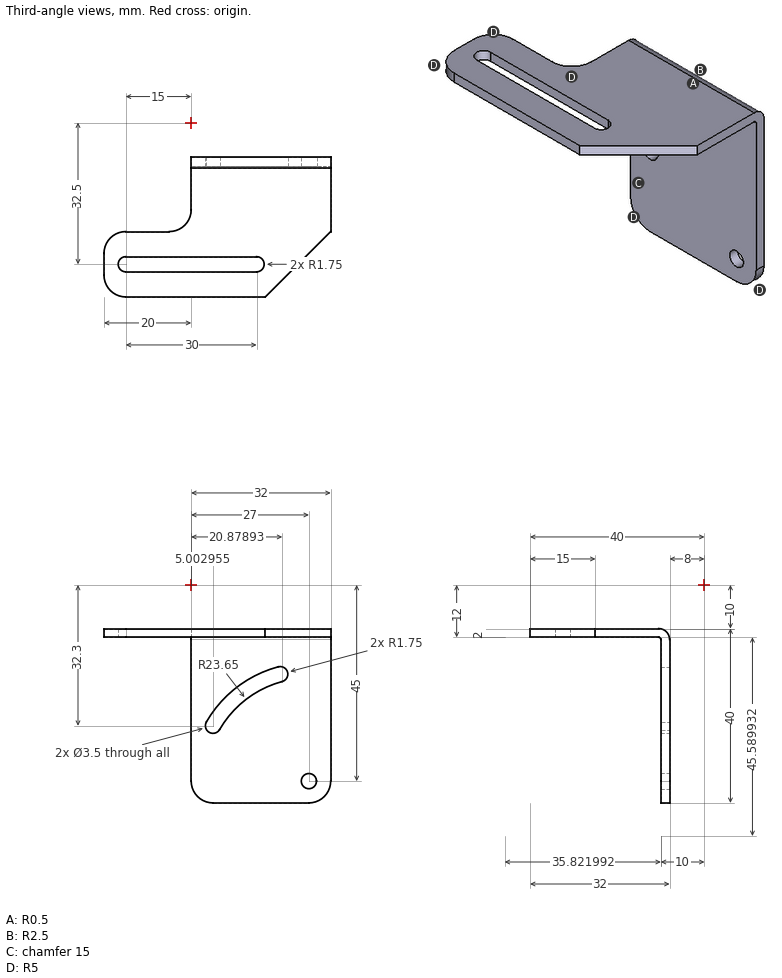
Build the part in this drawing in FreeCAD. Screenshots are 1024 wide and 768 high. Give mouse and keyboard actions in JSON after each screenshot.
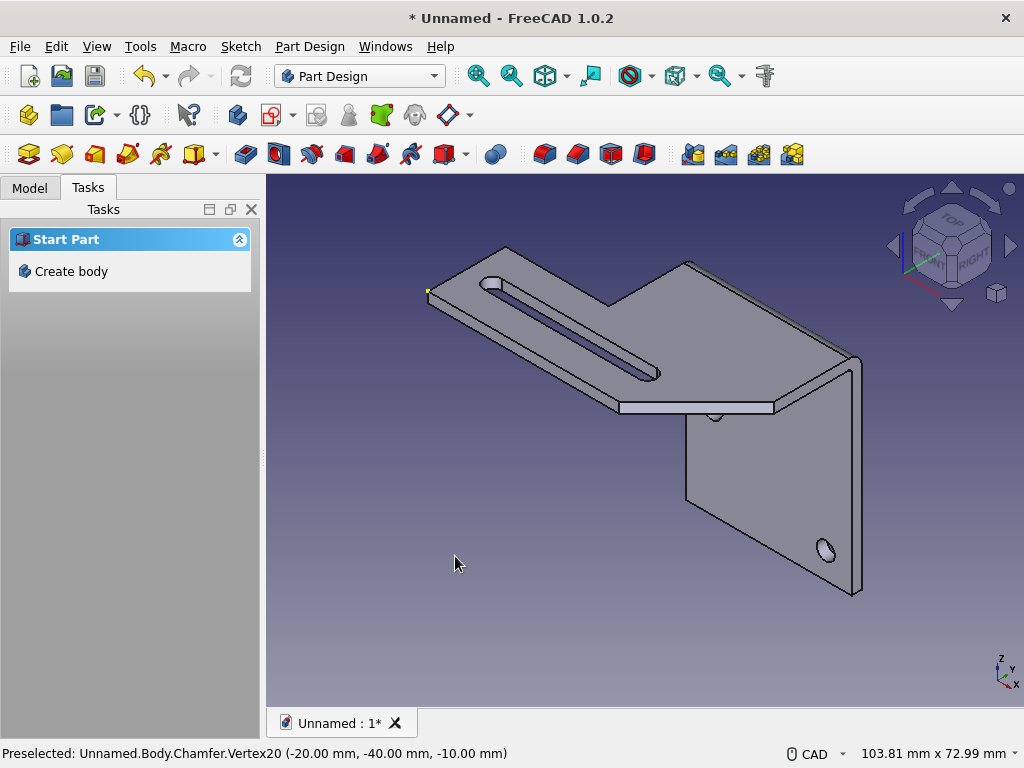
{"action": "scroll", "coordinate": [428, 296], "scroll_direction": "up", "scroll_amount": 6}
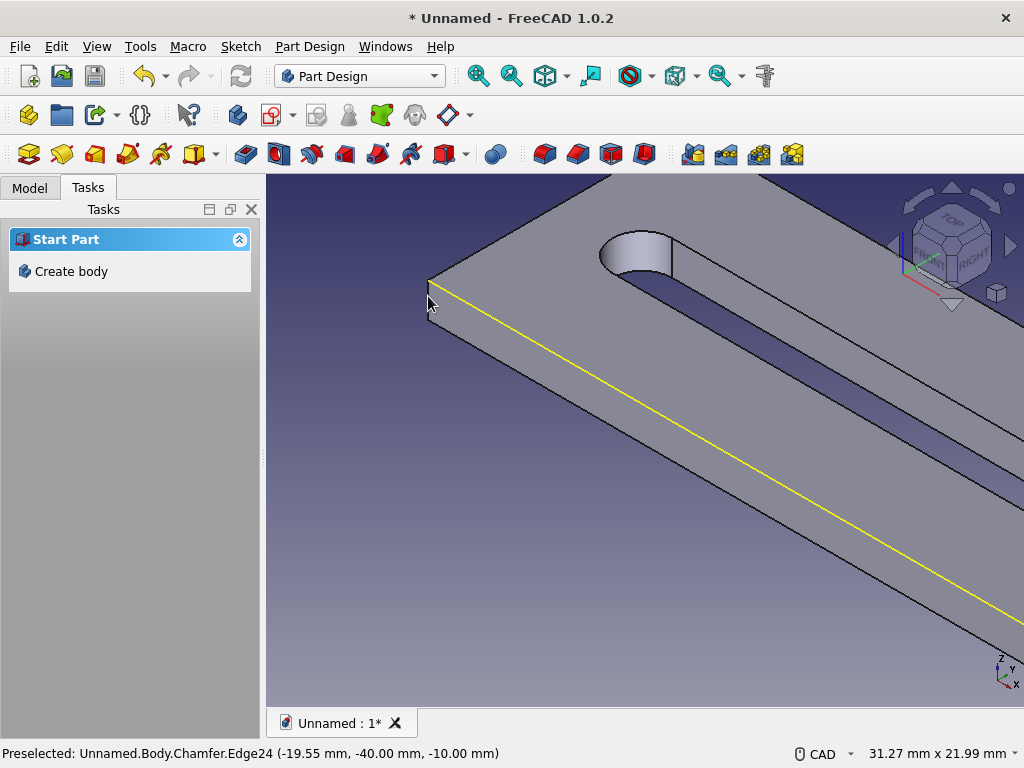
{"action": "left_click", "coordinate": [479, 76]}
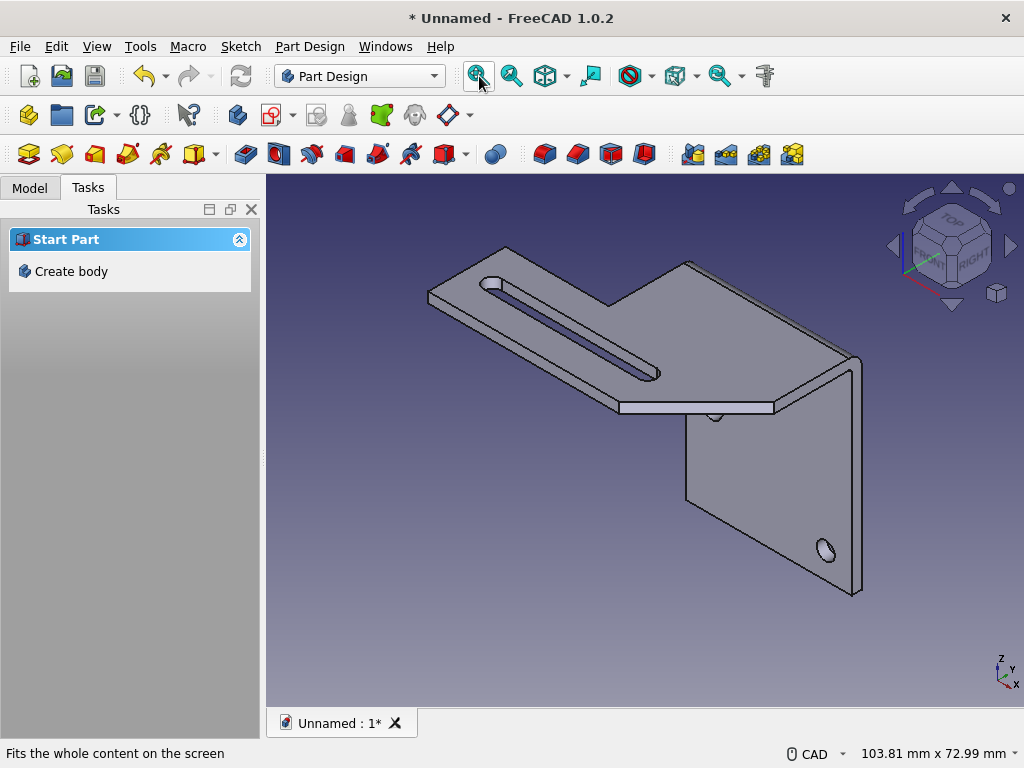
{"action": "key", "text": "1"}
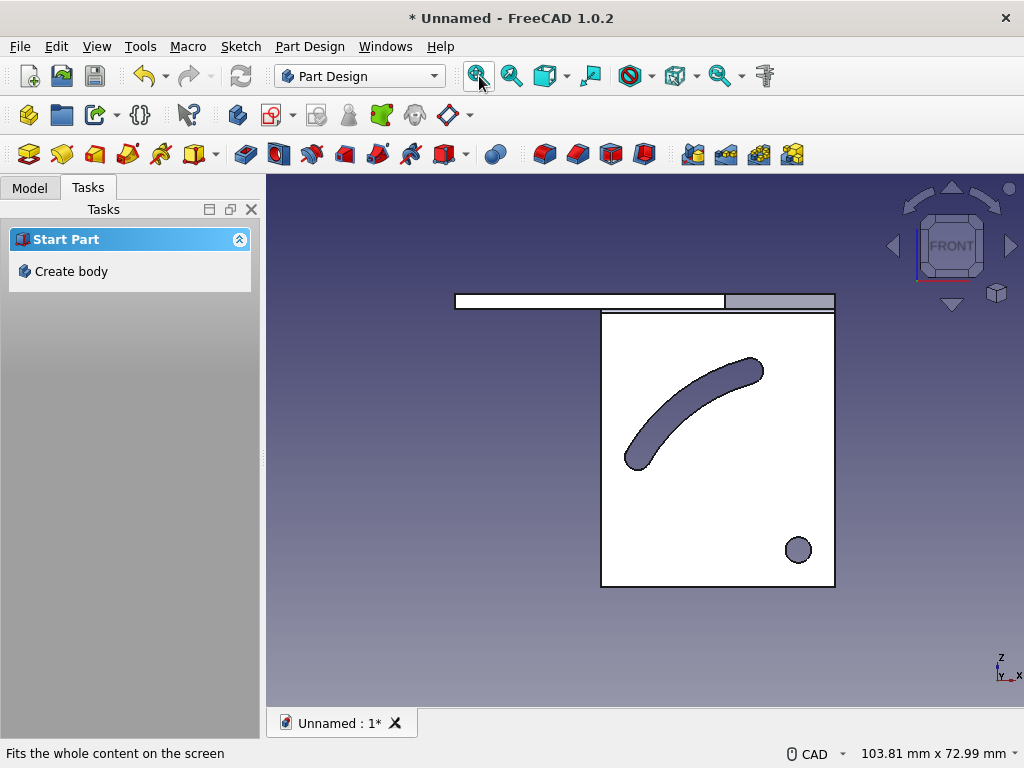
{"action": "left_click", "coordinate": [455, 301]}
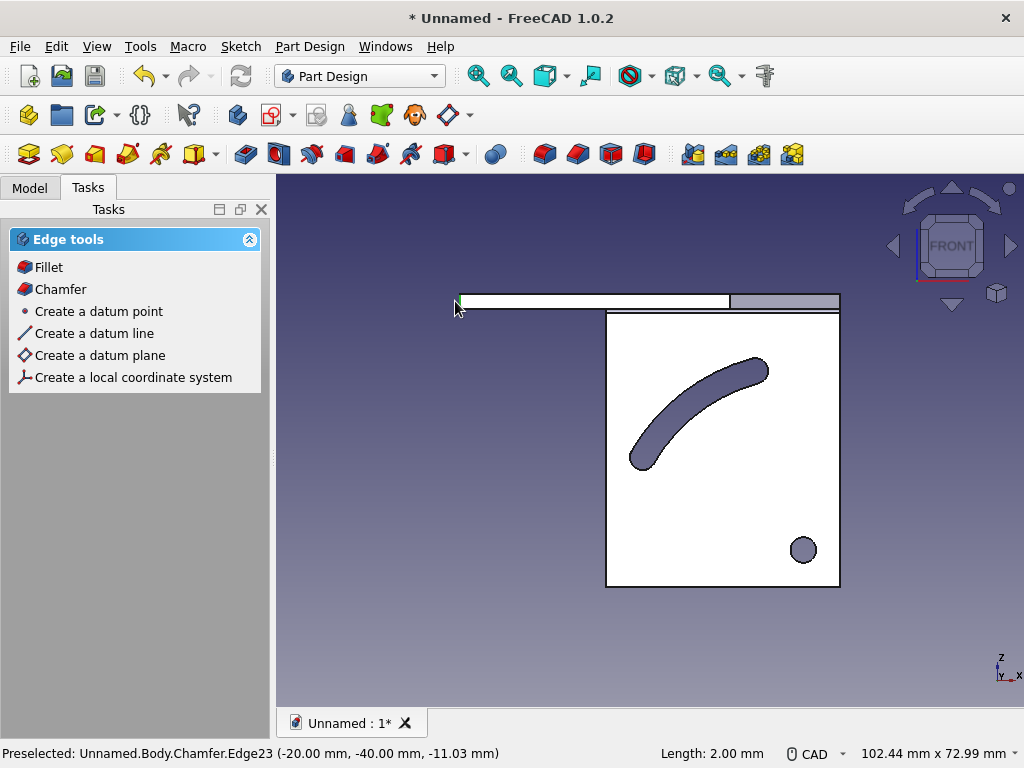
{"action": "scroll", "coordinate": [606, 301], "scroll_direction": "up", "scroll_amount": 6}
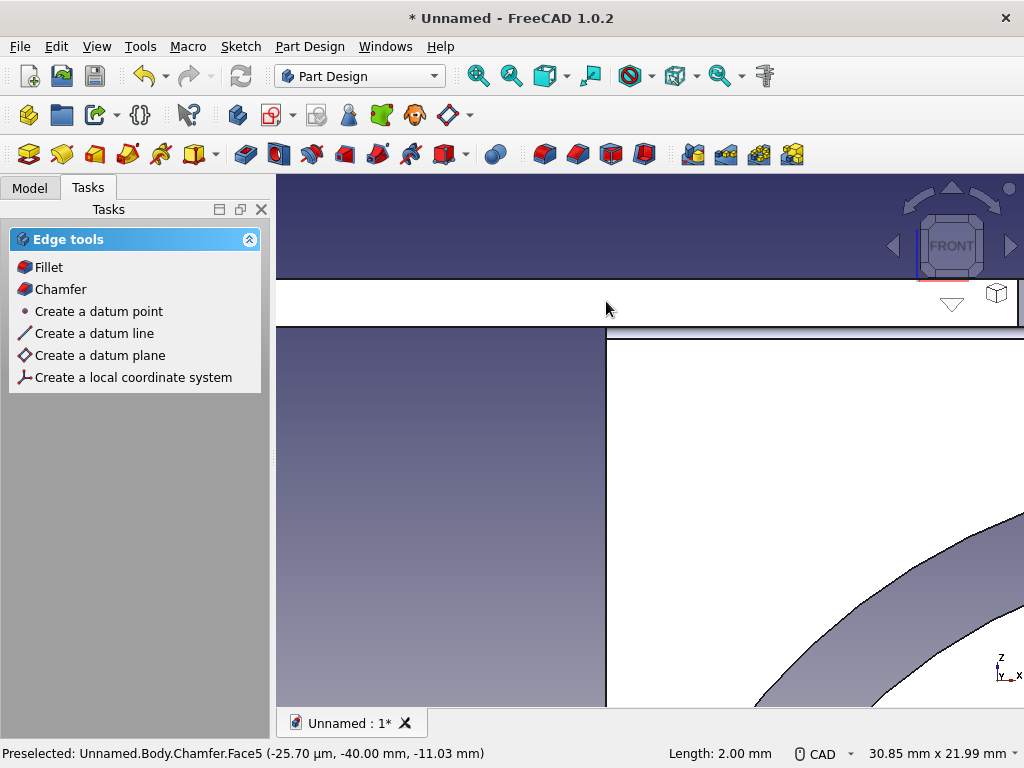
{"action": "key", "text": "v f"}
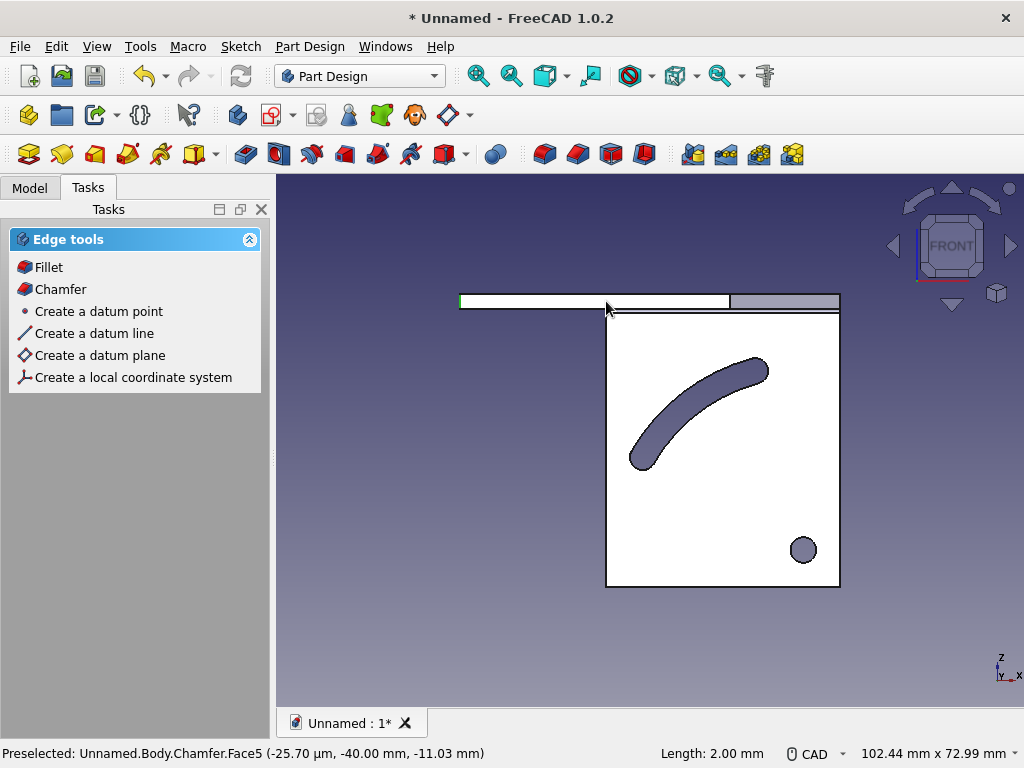
{"action": "key", "text": "3"}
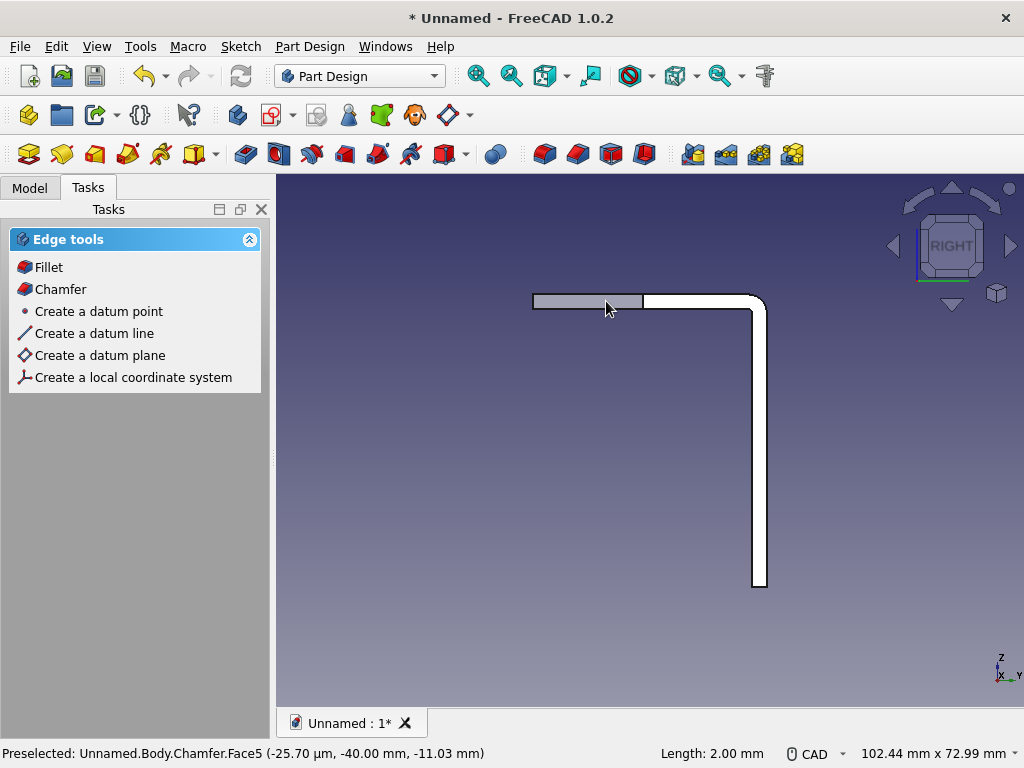
{"action": "left_click", "coordinate": [760, 586], "text": "ctrl"}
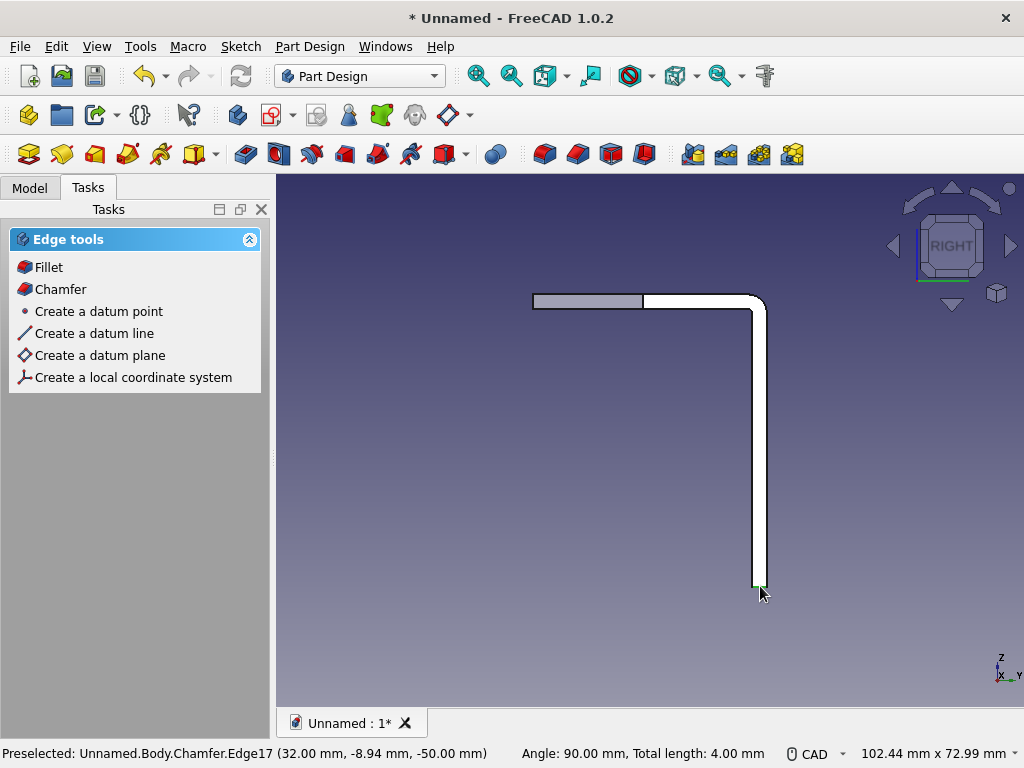
{"action": "scroll", "coordinate": [643, 301], "scroll_direction": "up", "scroll_amount": 6}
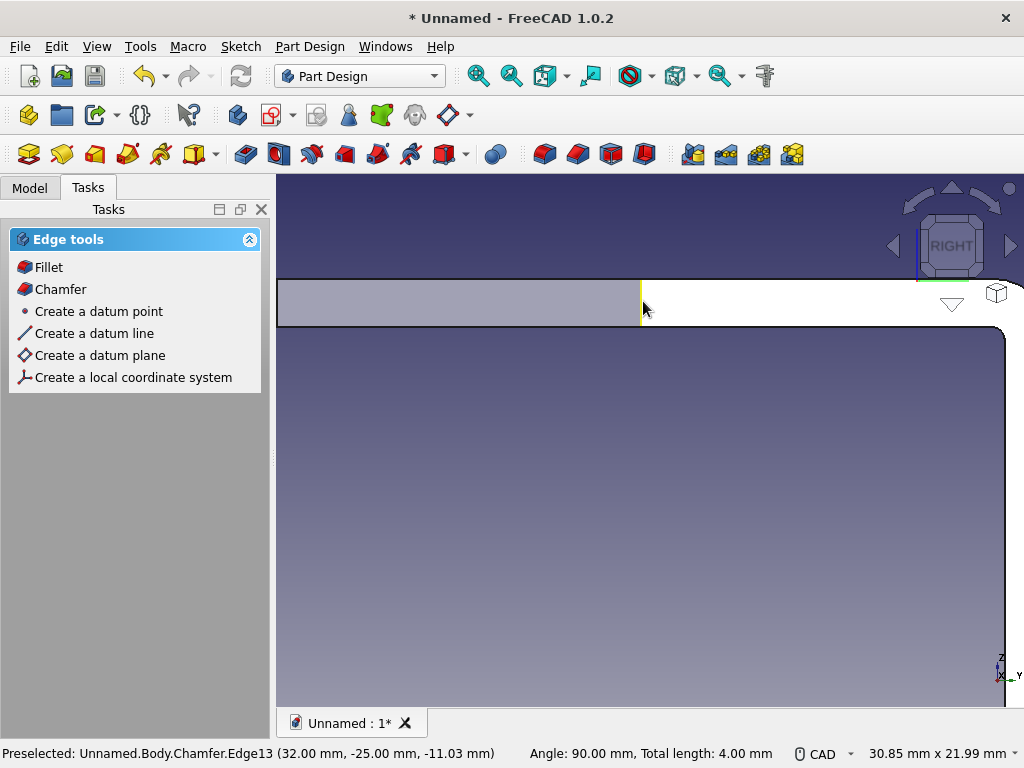
{"action": "left_click", "coordinate": [479, 76]}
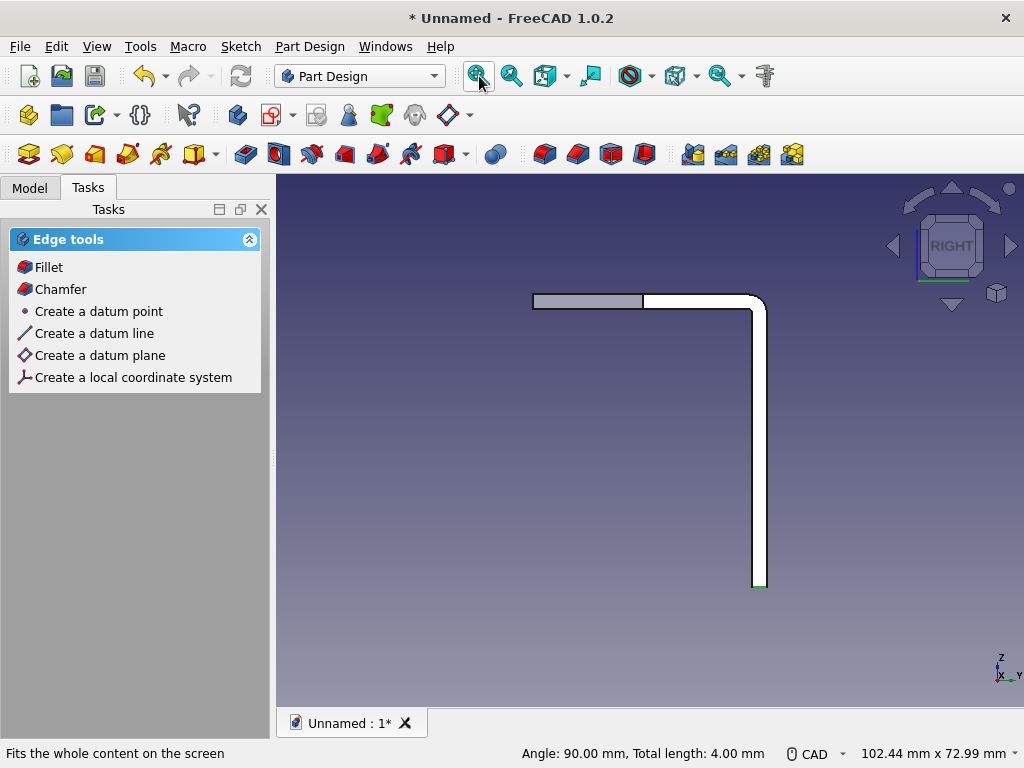
{"action": "key", "text": "5"}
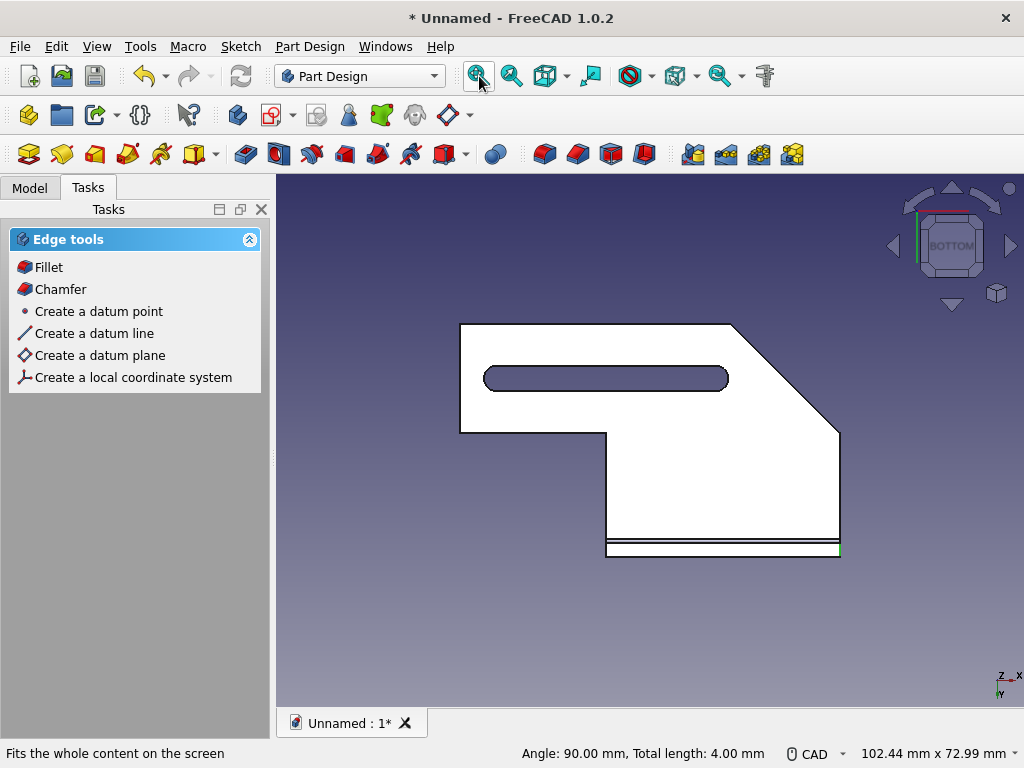
{"action": "left_click", "coordinate": [606, 549], "text": "ctrl"}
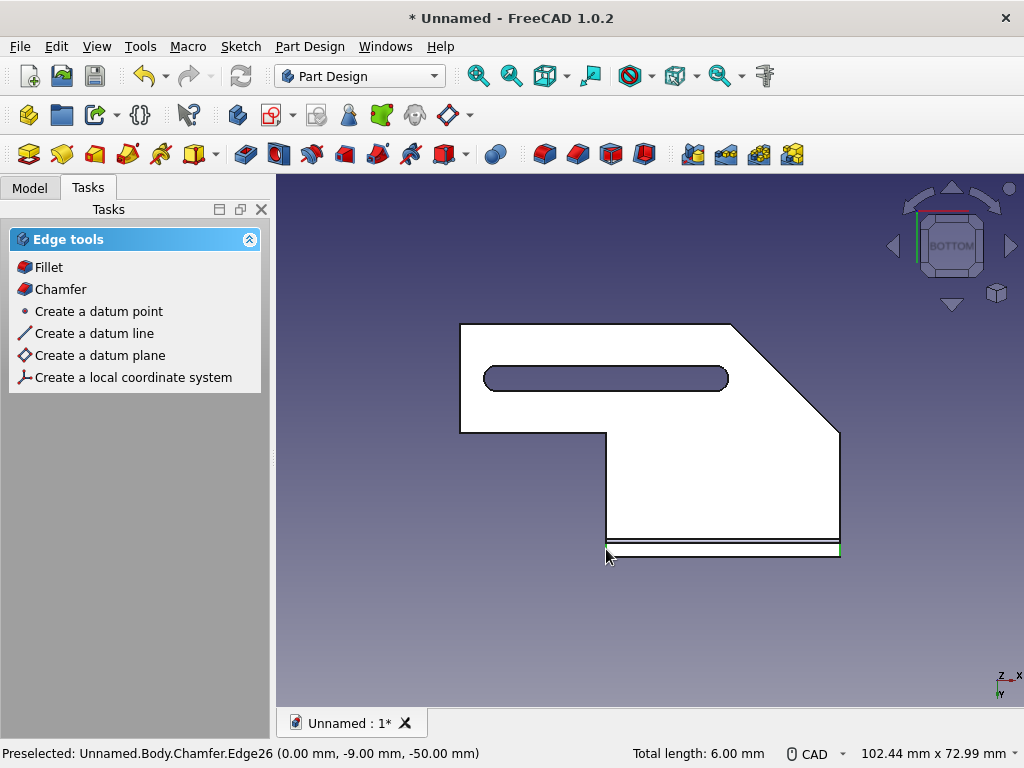
{"action": "scroll", "coordinate": [606, 432], "scroll_direction": "up", "scroll_amount": 6}